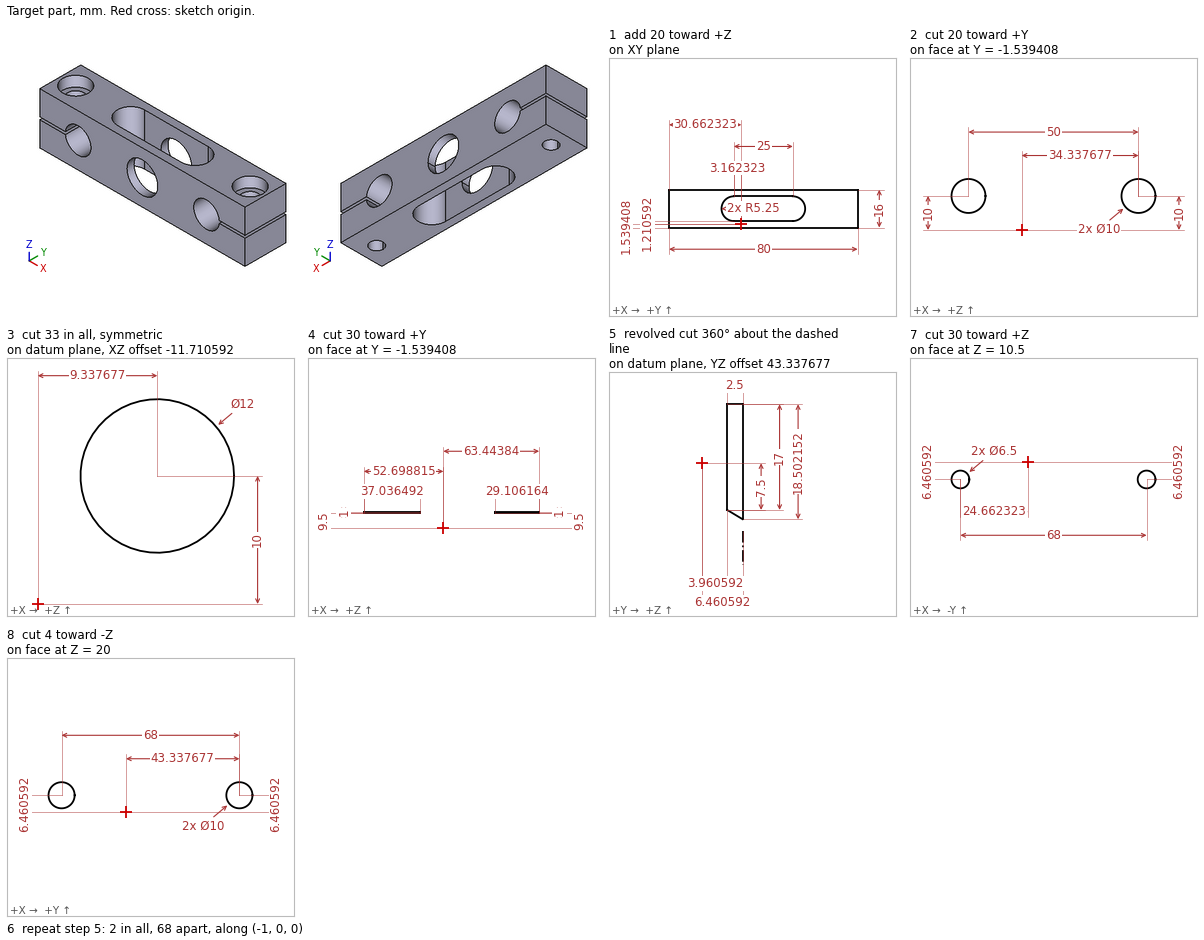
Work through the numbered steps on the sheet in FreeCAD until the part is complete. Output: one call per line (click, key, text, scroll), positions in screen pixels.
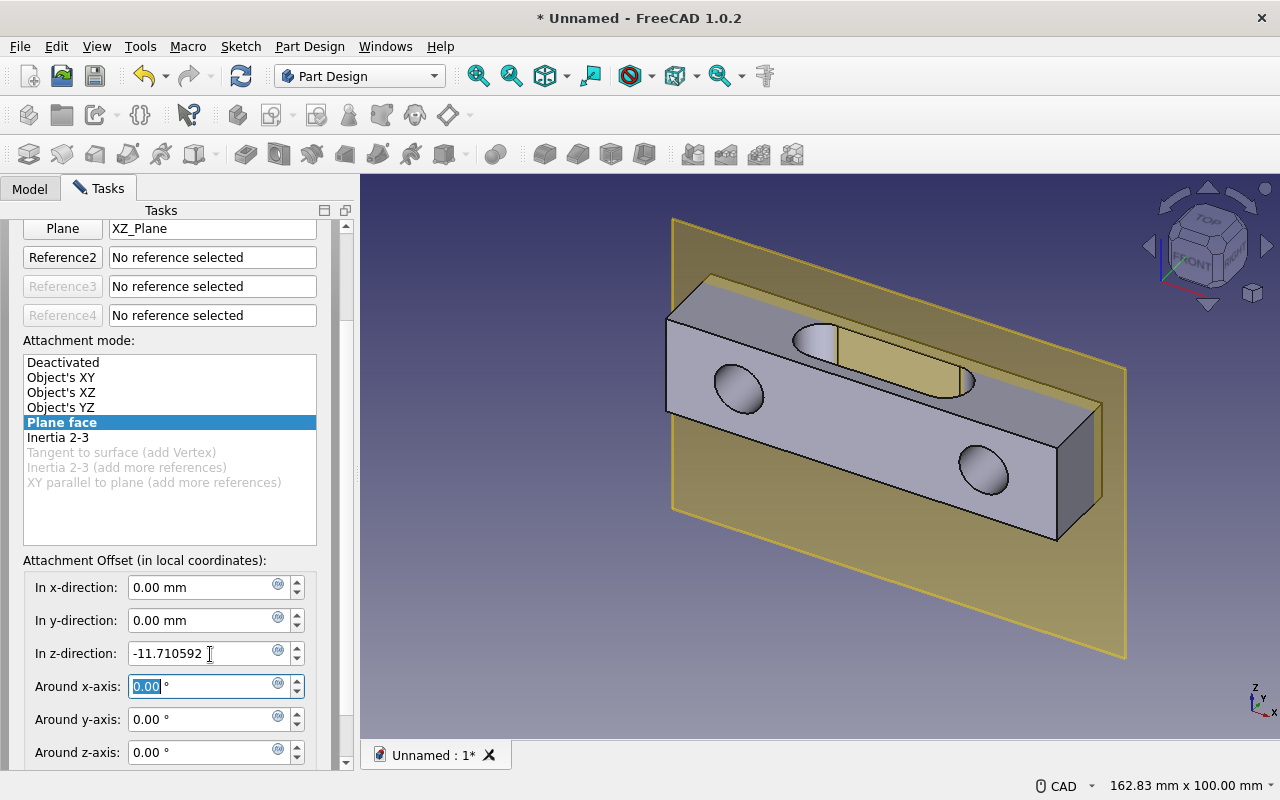
scroll(346, 495, up, 3)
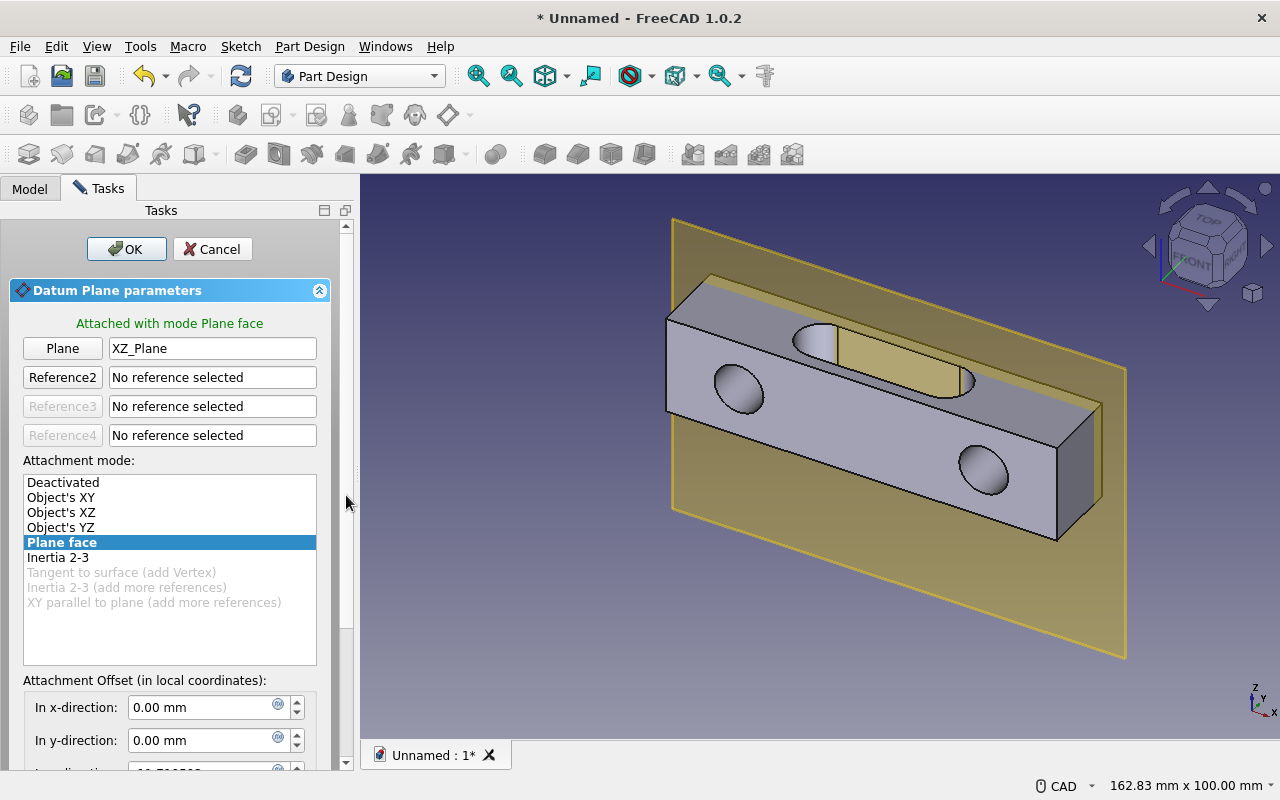
click(127, 249)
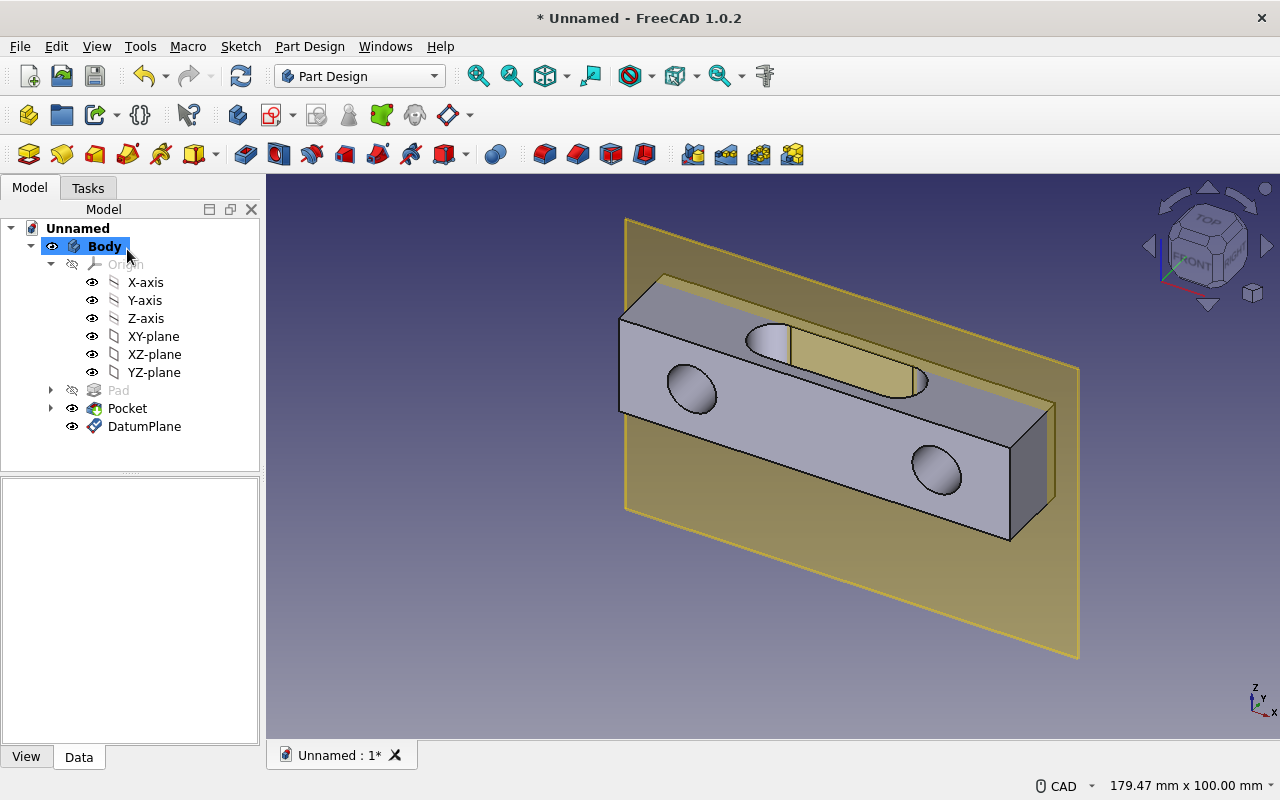
click(117, 426)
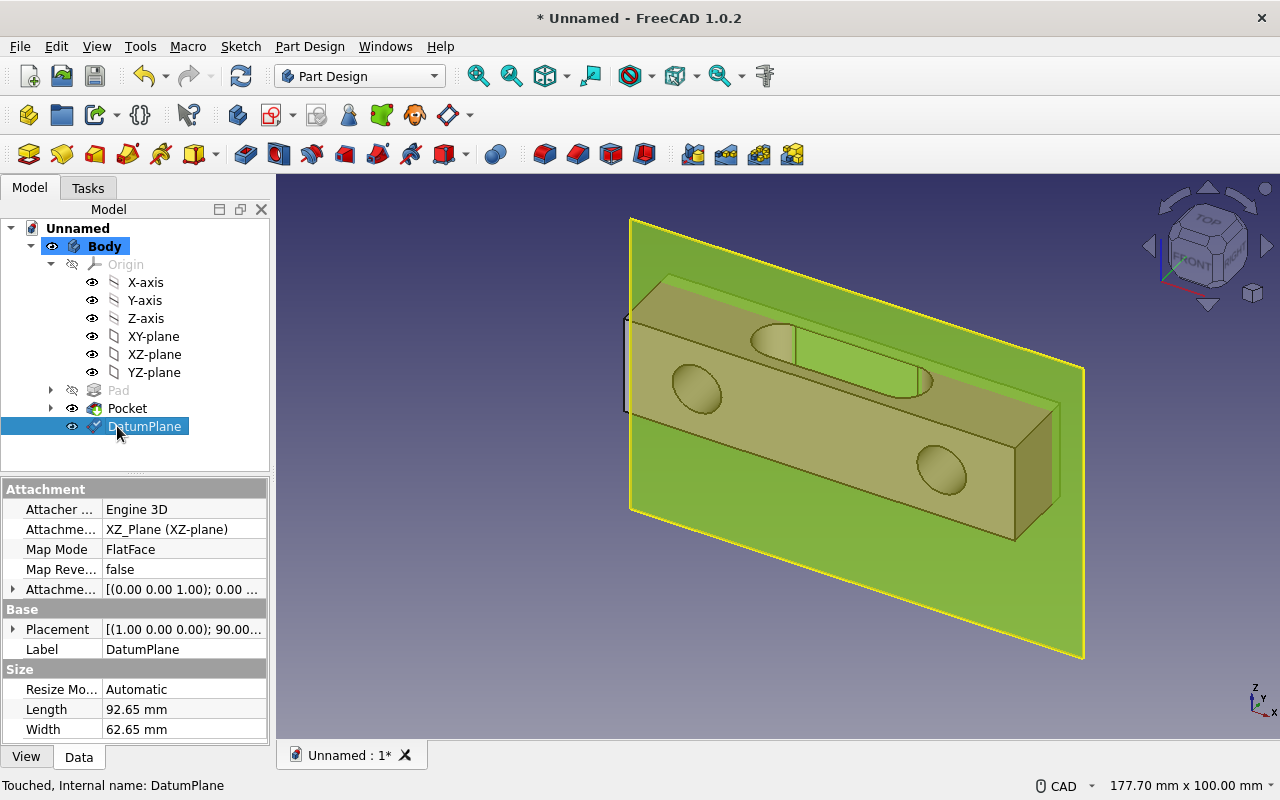
click(270, 116)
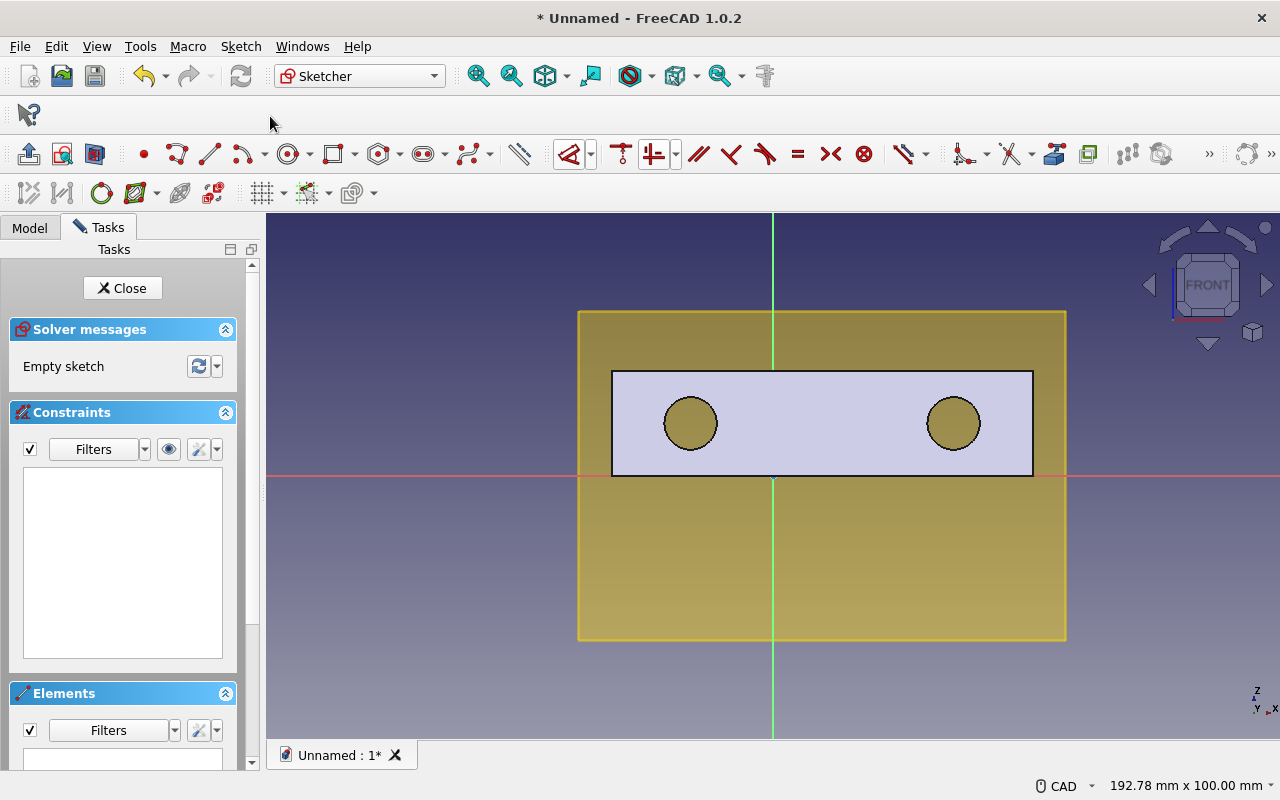
click(95, 154)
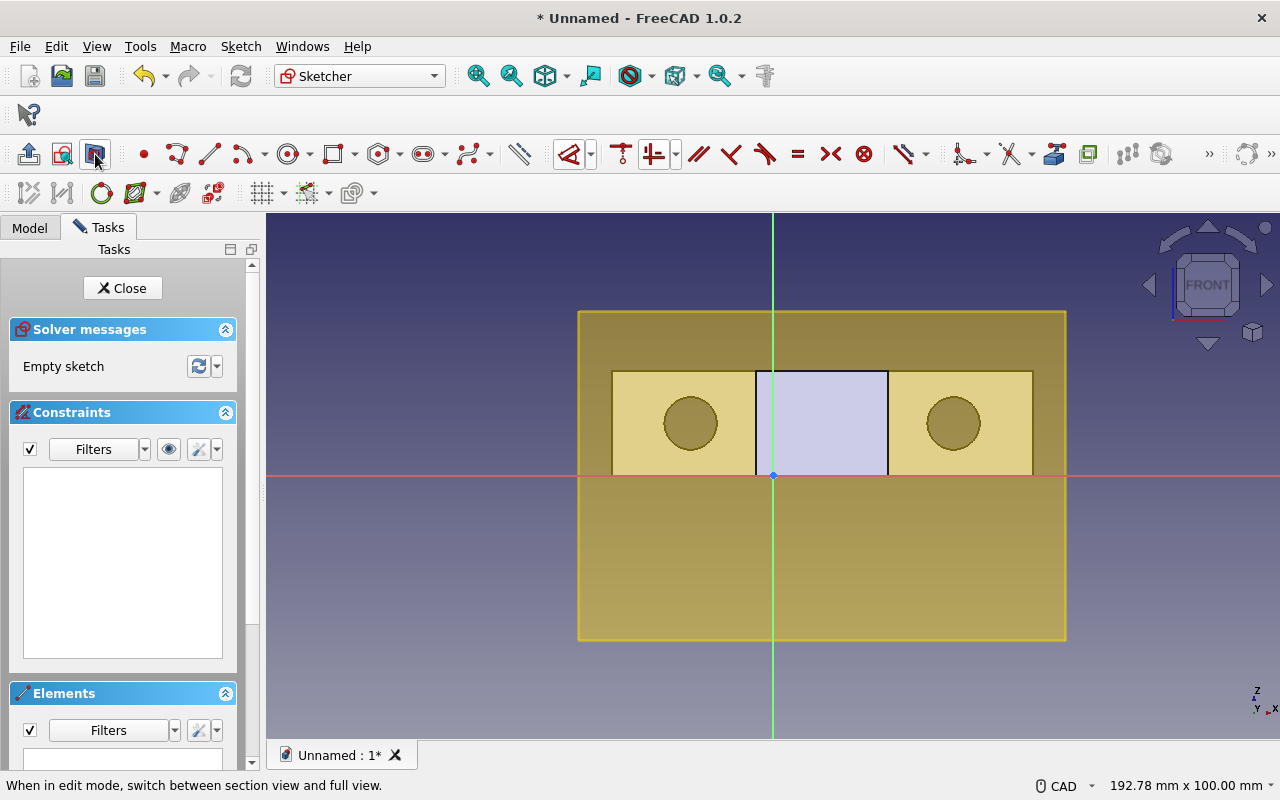
scroll(849, 420, up, 7)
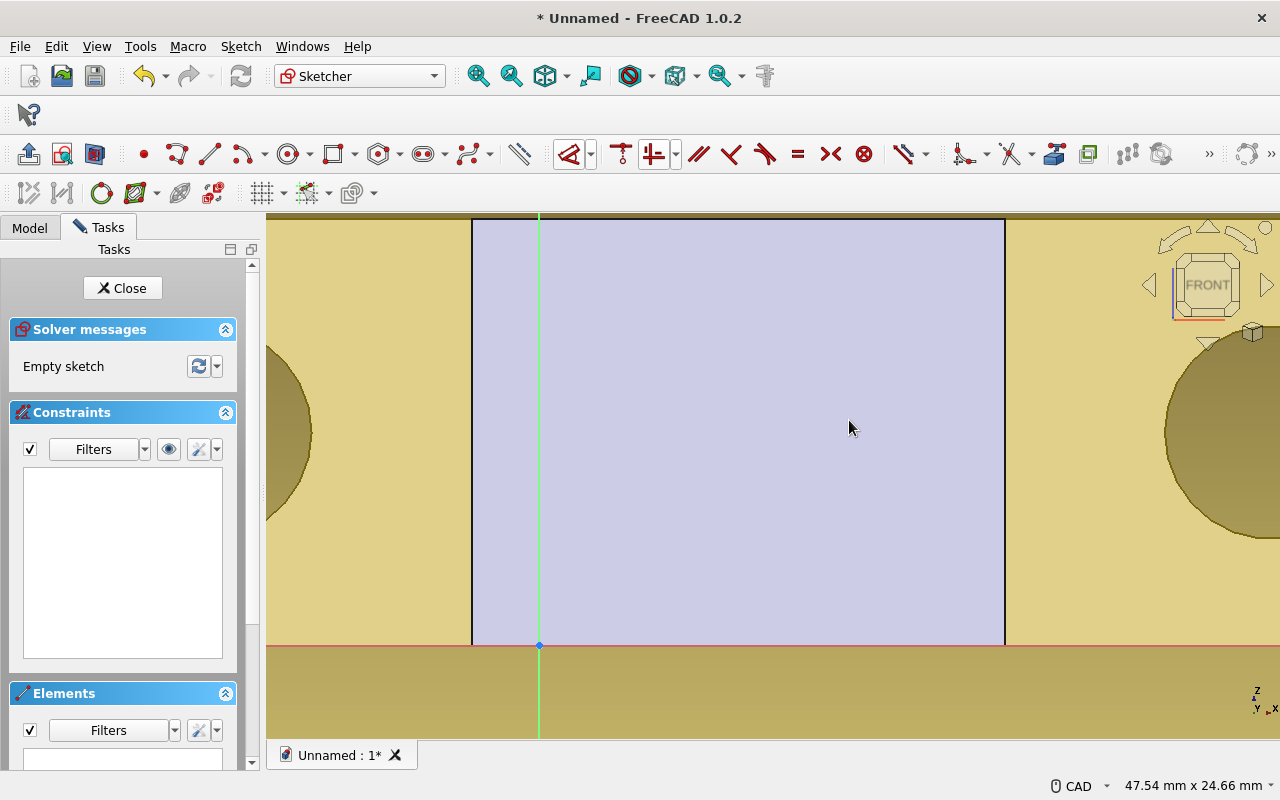
click(288, 154)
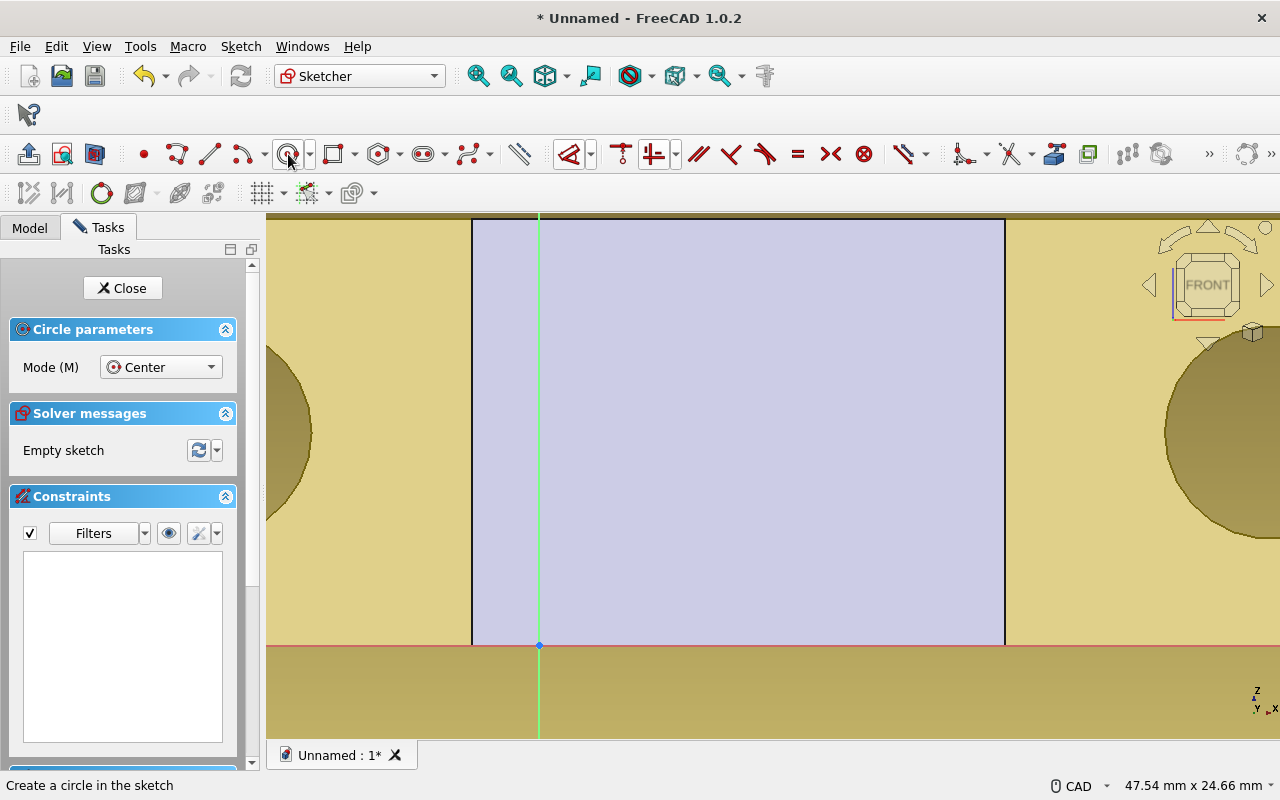
click(738, 433)
move(829, 342)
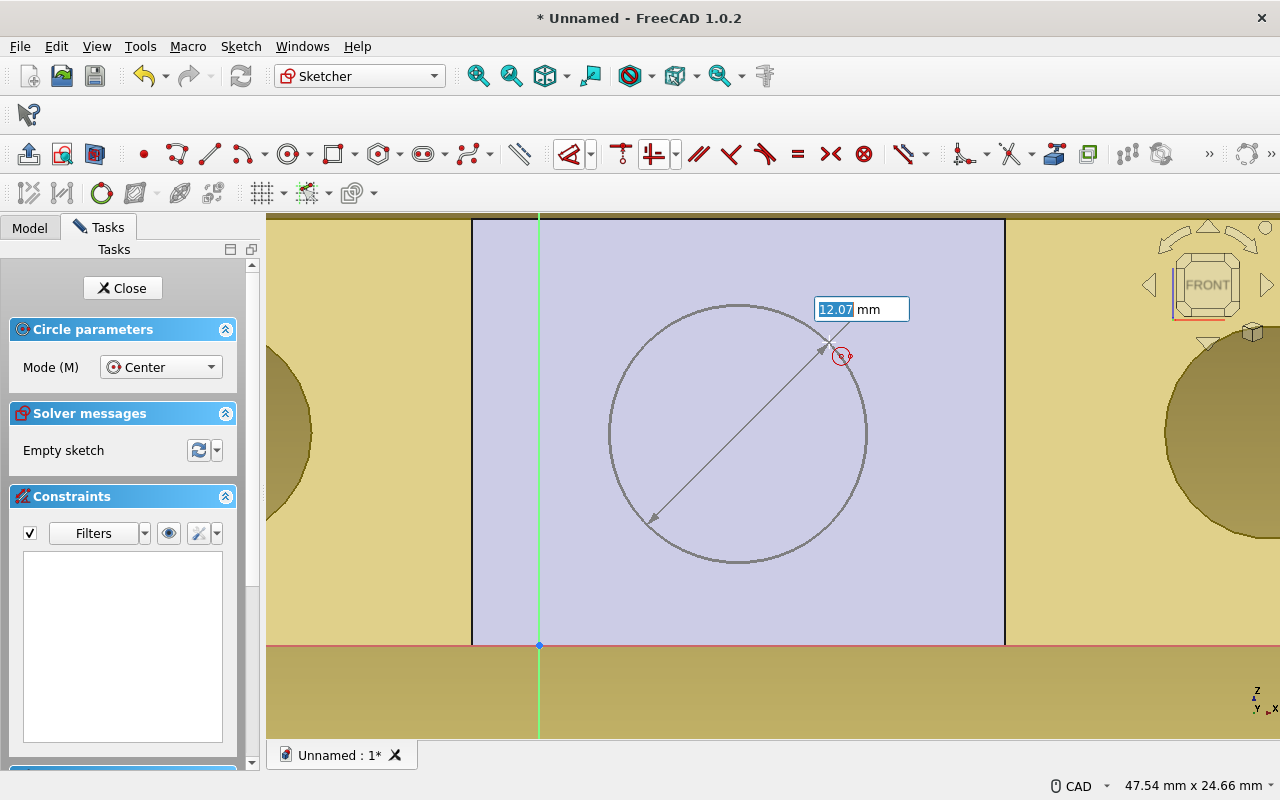
text(12)
key(Return)
key(Escape)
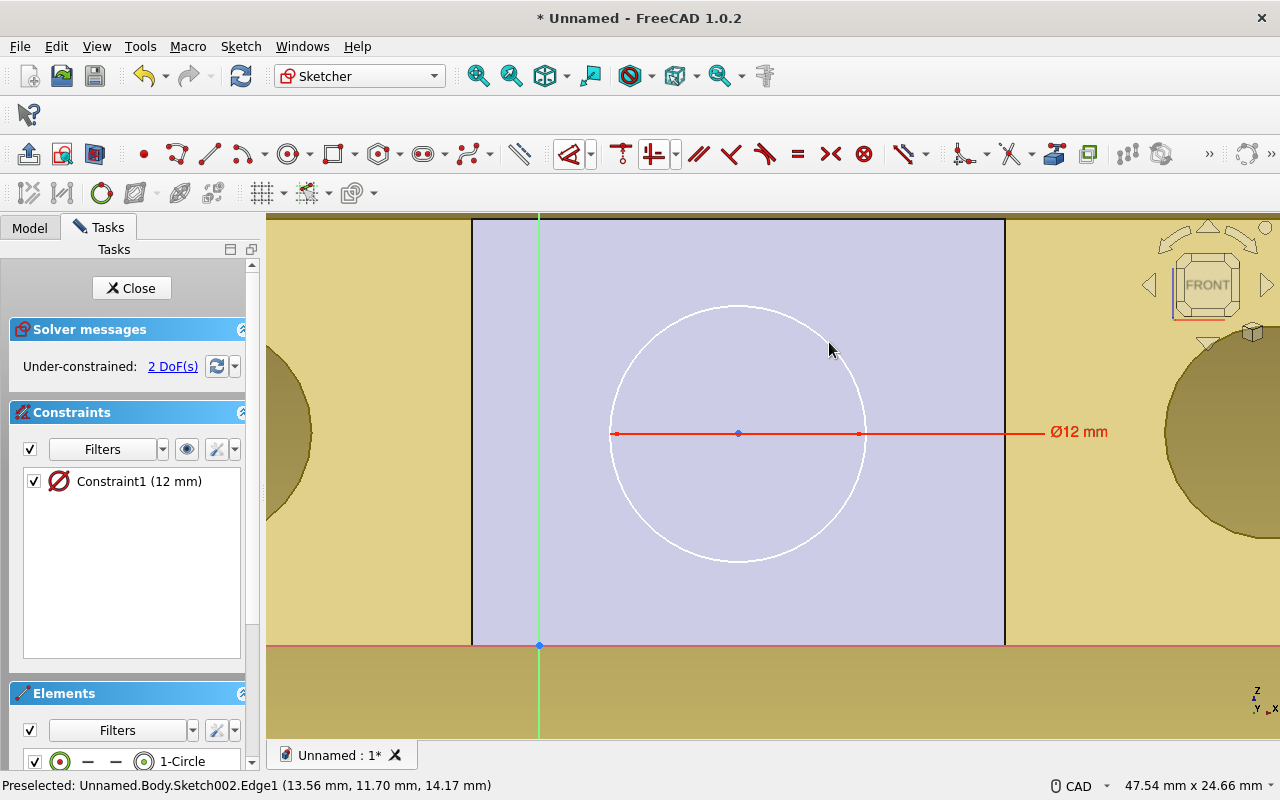
click(738, 434)